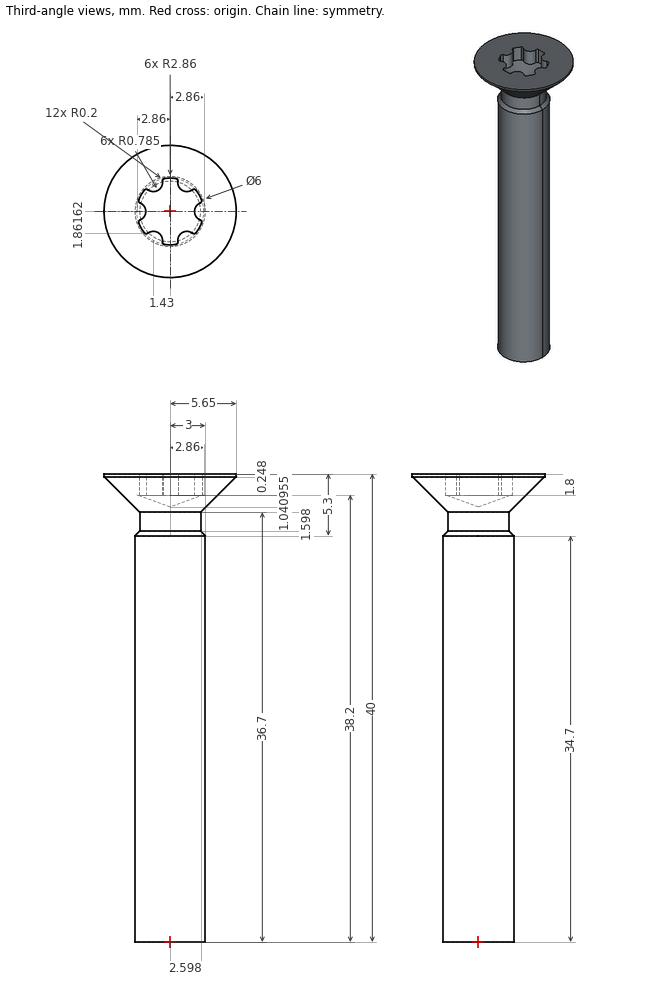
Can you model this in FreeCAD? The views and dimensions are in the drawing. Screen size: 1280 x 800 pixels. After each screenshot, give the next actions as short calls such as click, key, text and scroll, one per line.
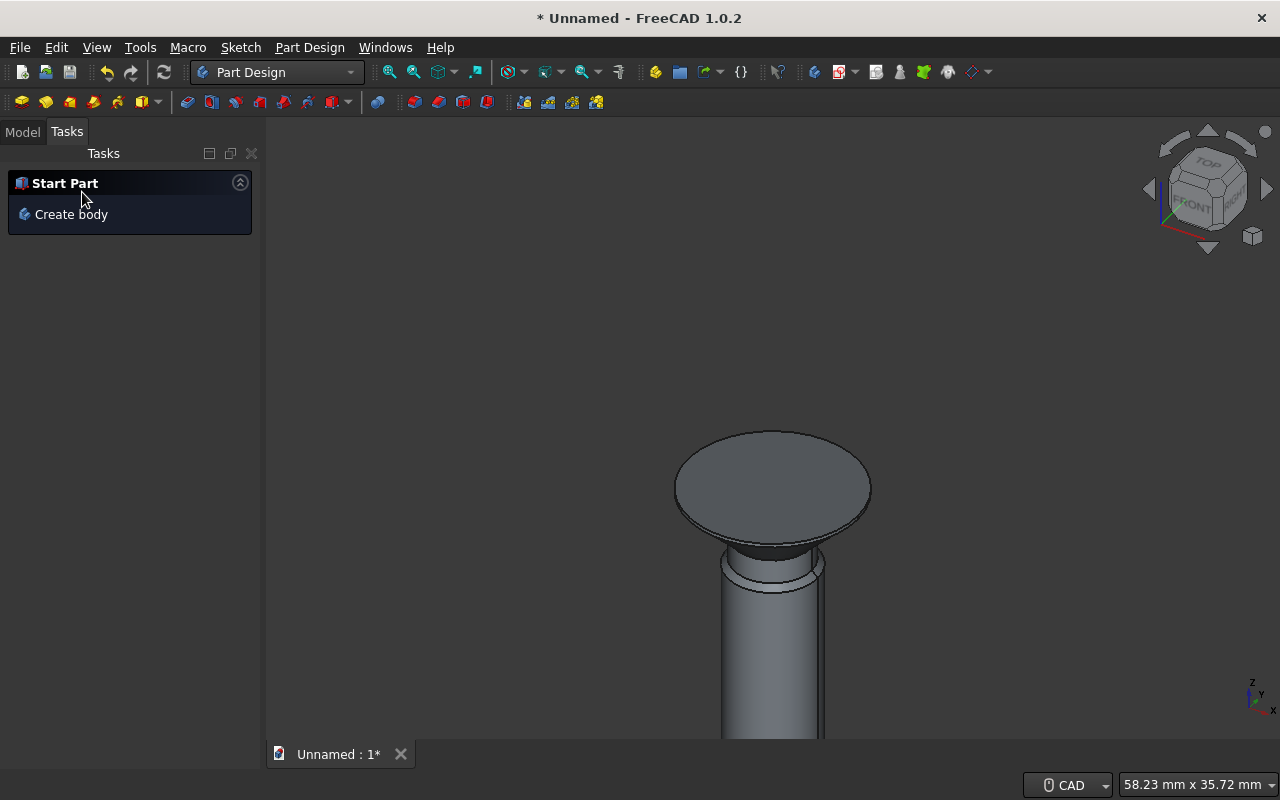
click(390, 72)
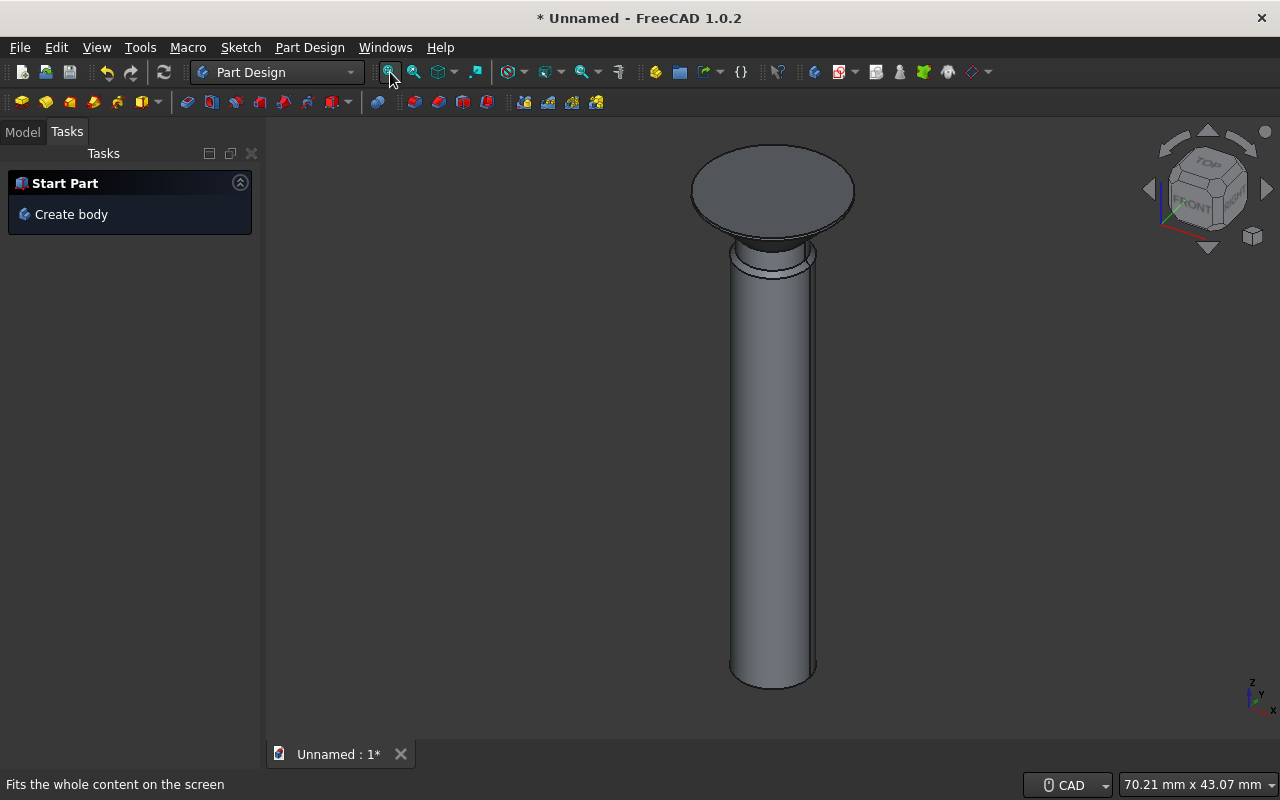
click(773, 190)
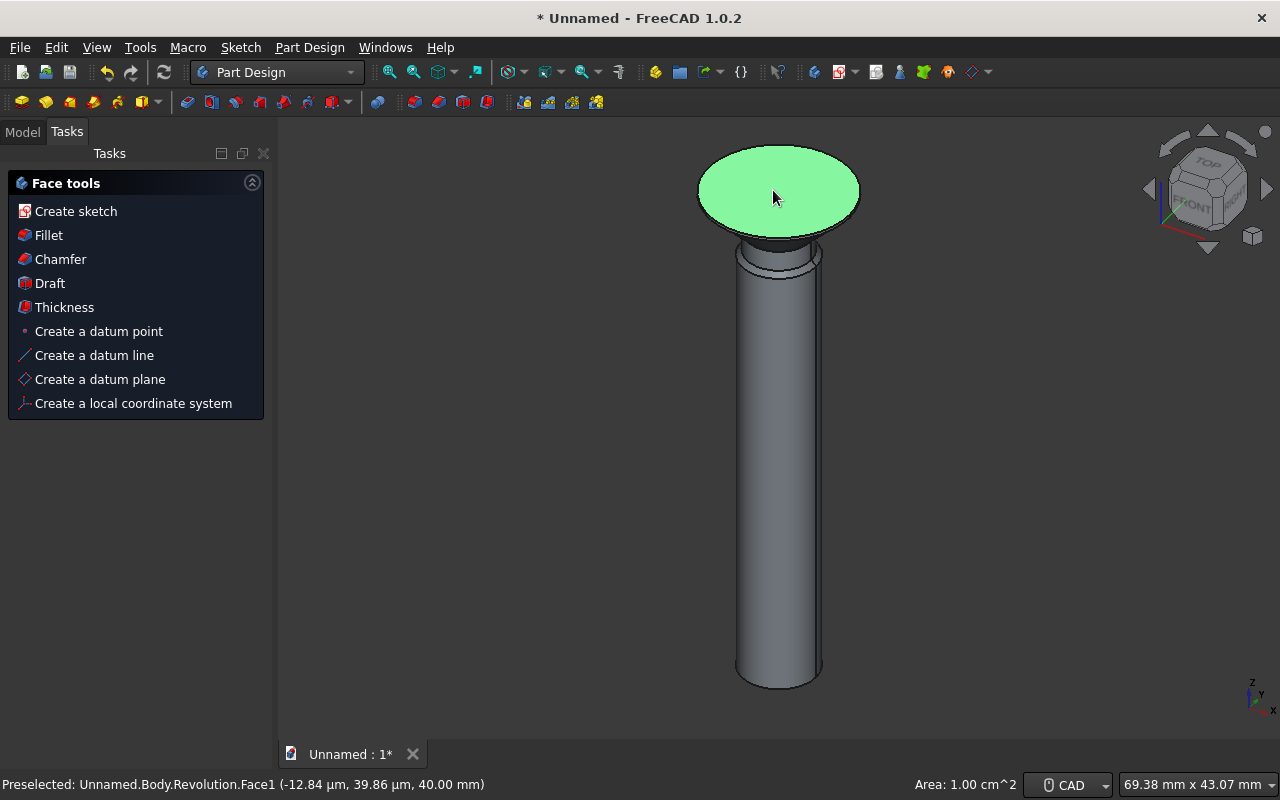
click(840, 72)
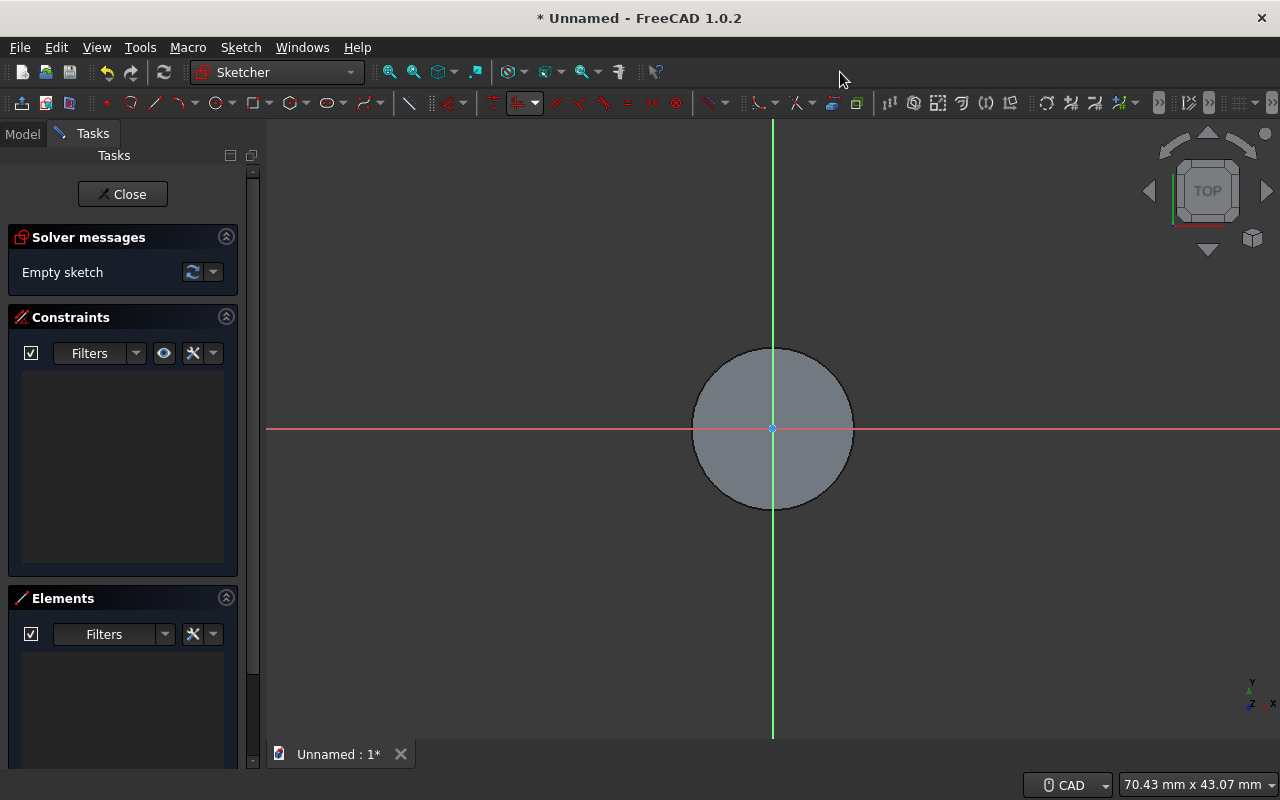
scroll(790, 429, up, 8)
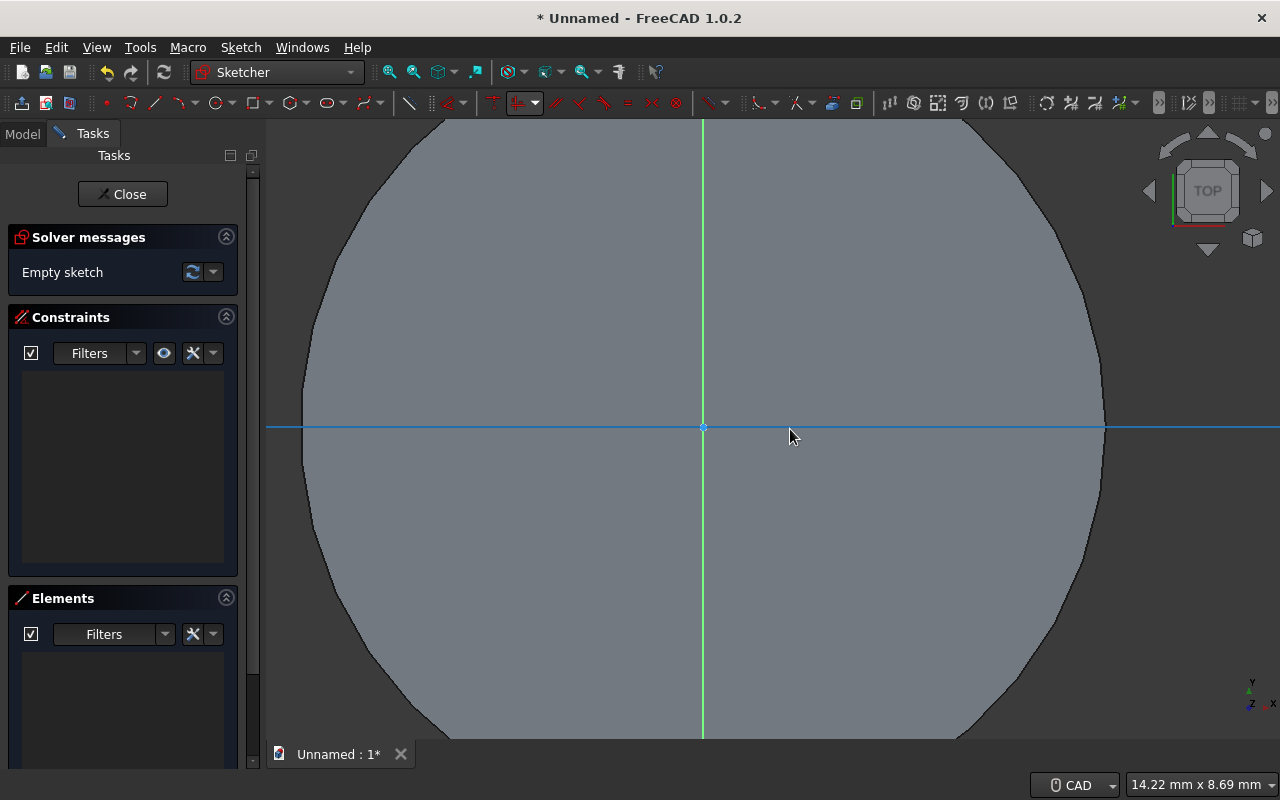
click(180, 104)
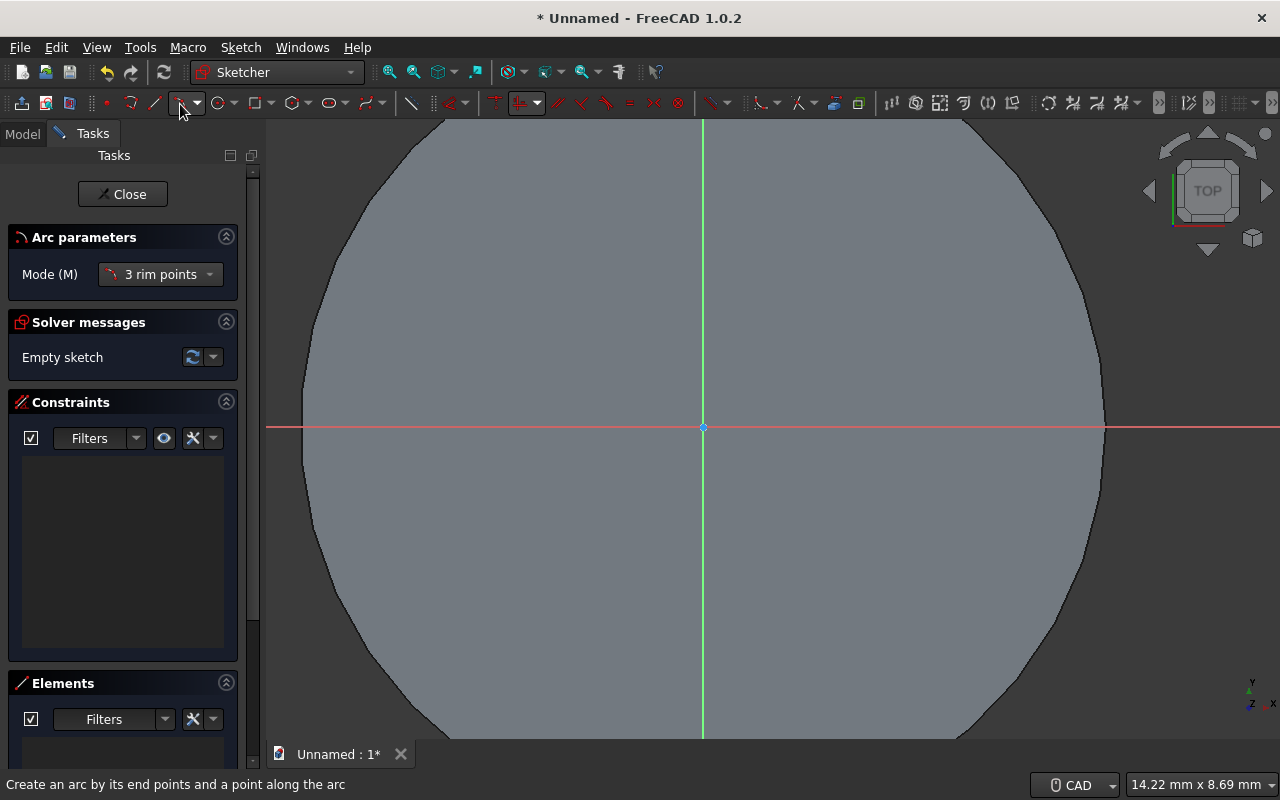
click(520, 375)
click(520, 479)
click(549, 453)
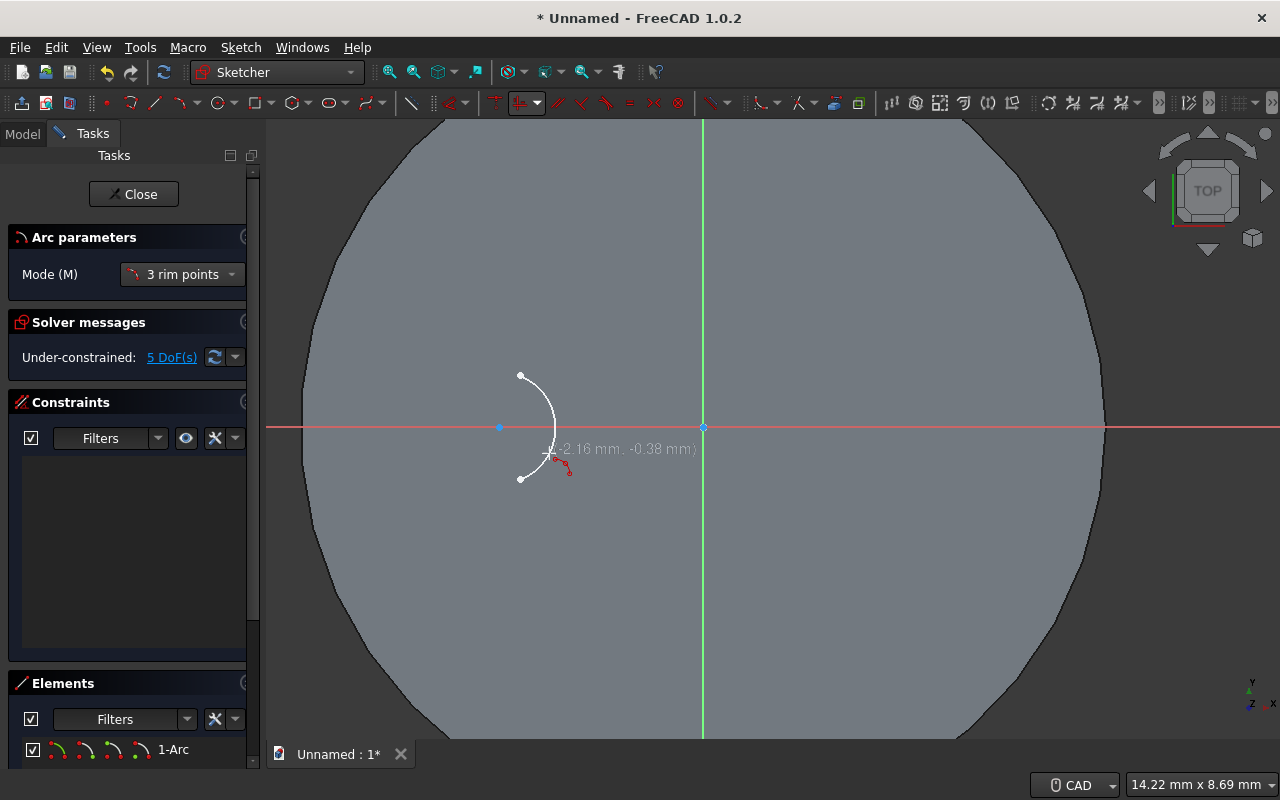
click(520, 480)
click(512, 497)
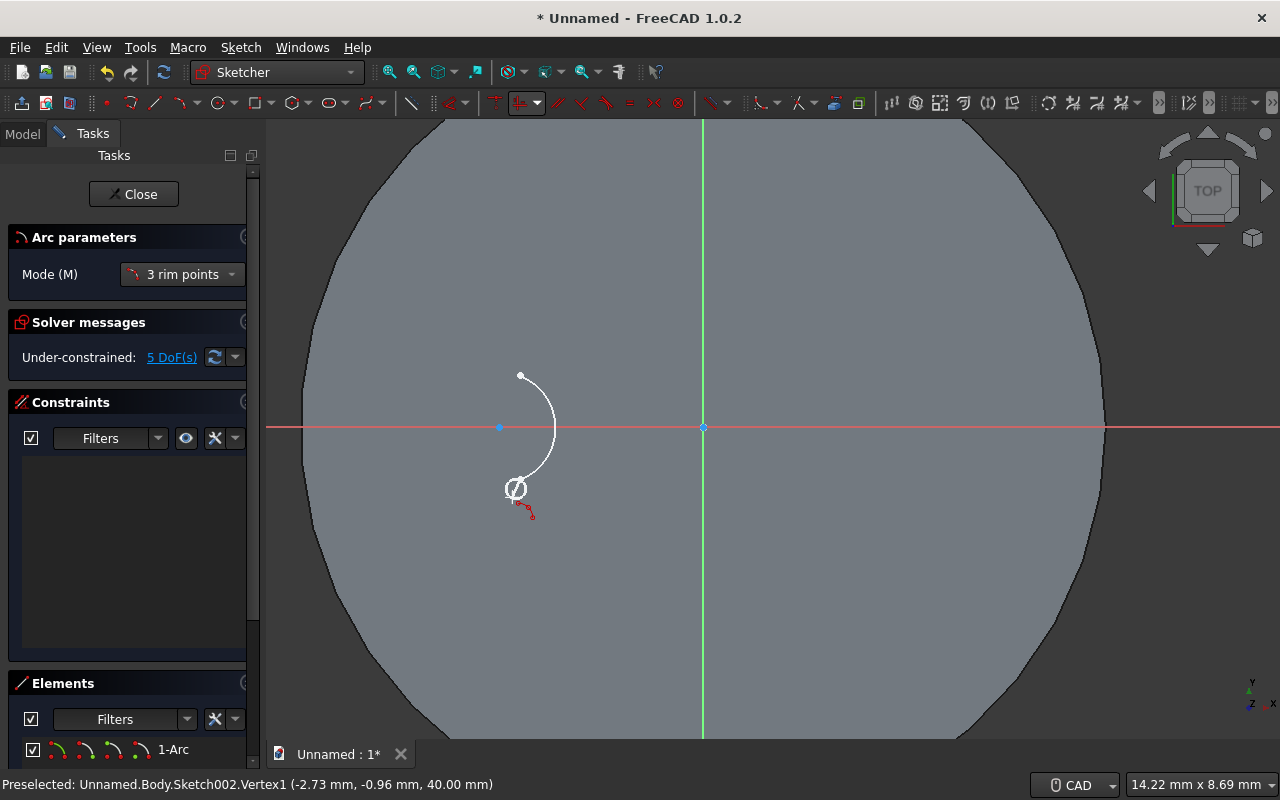
scroll(512, 486, up, 7)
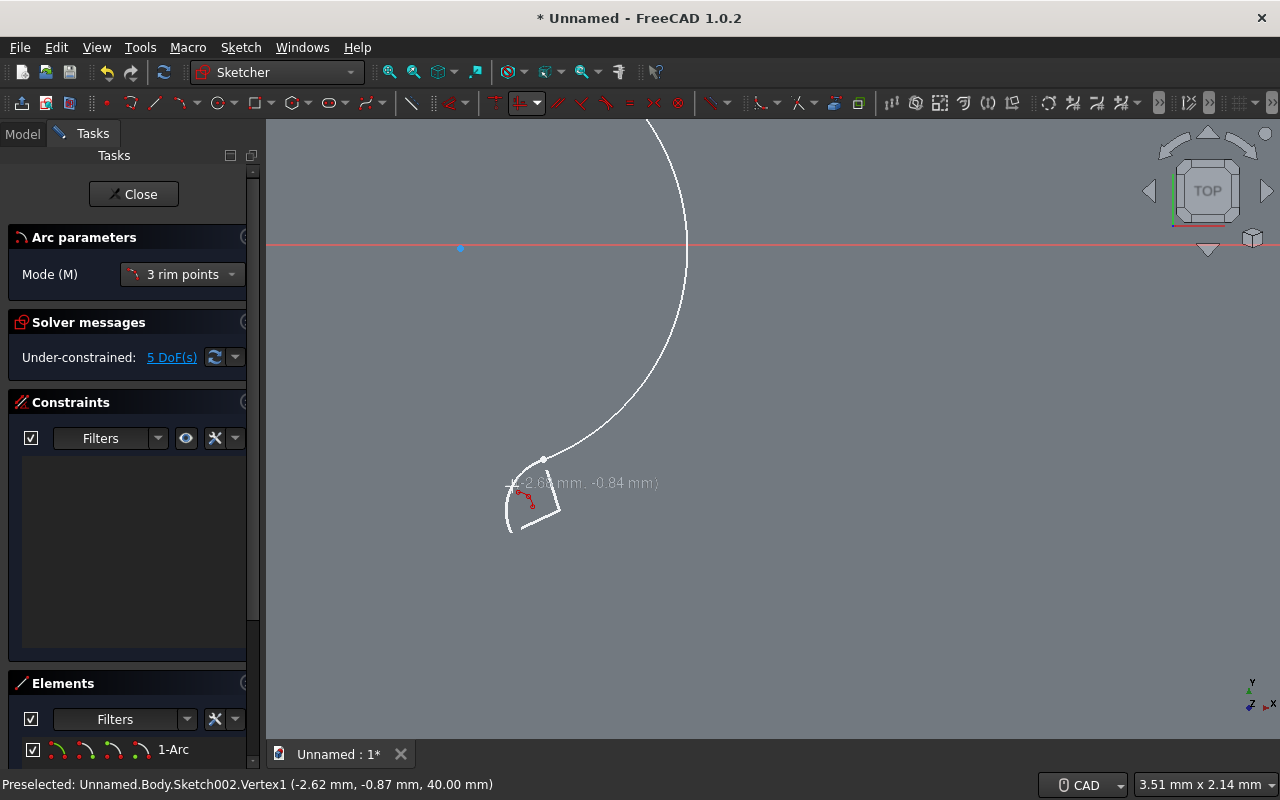
click(511, 486)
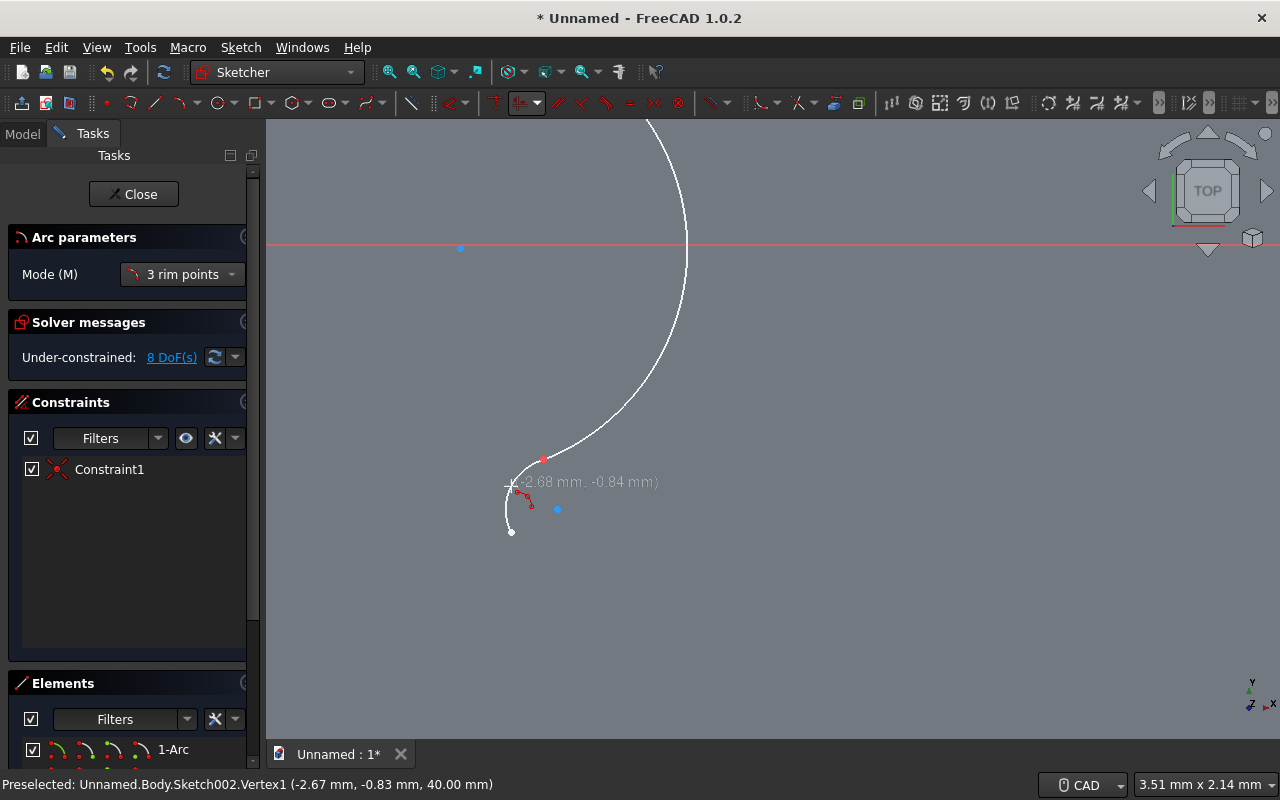
scroll(514, 489, down, 7)